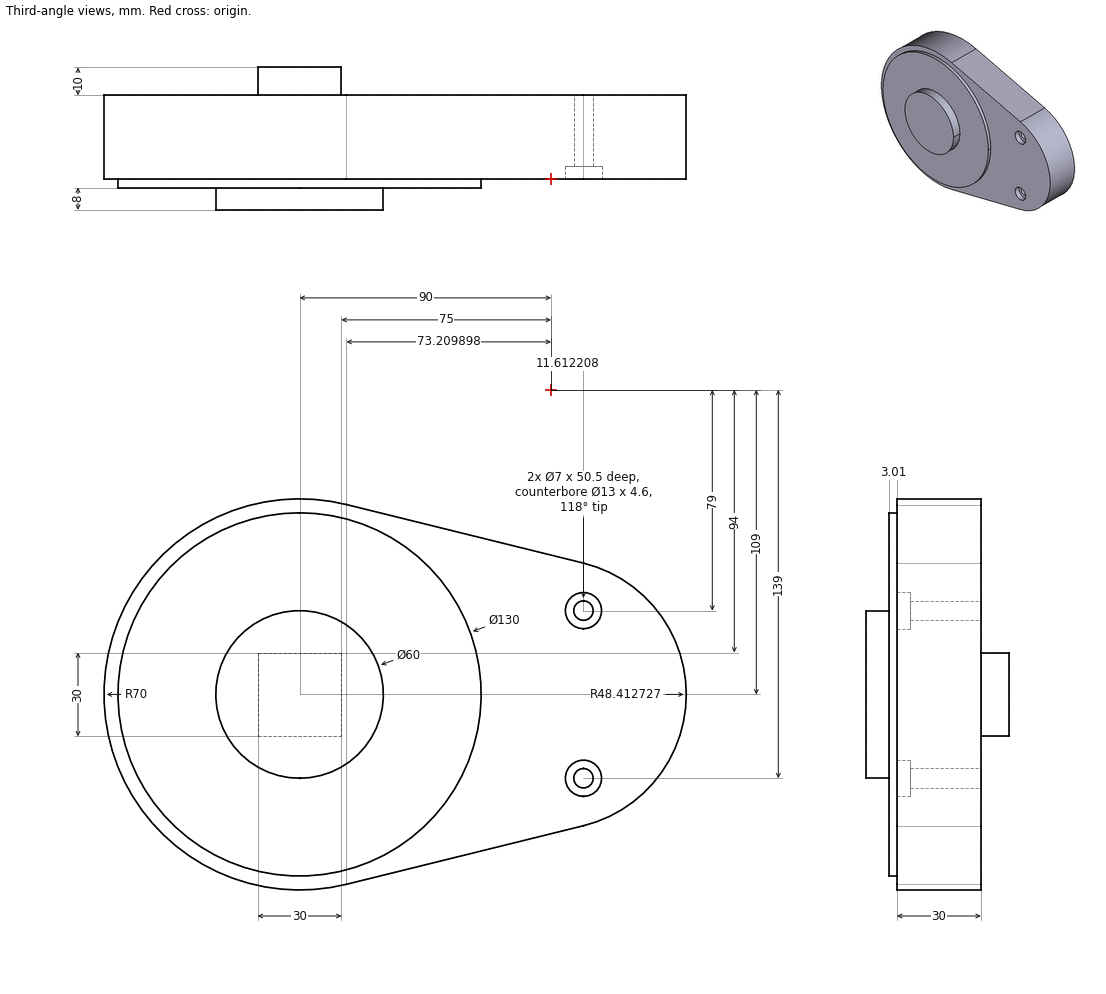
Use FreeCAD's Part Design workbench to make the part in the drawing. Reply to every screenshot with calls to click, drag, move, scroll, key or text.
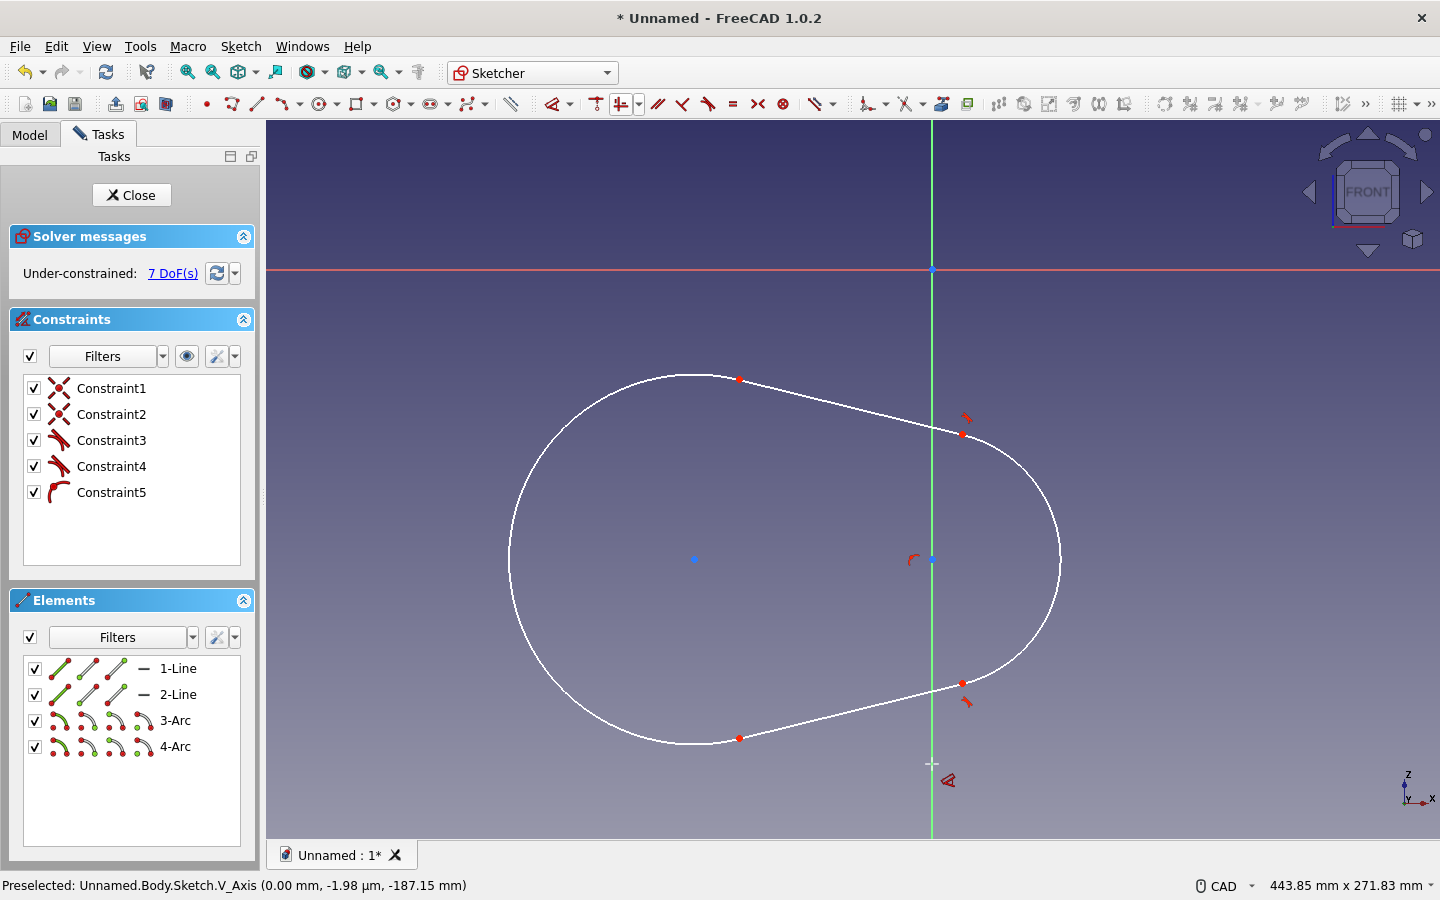
click(556, 437)
click(532, 416)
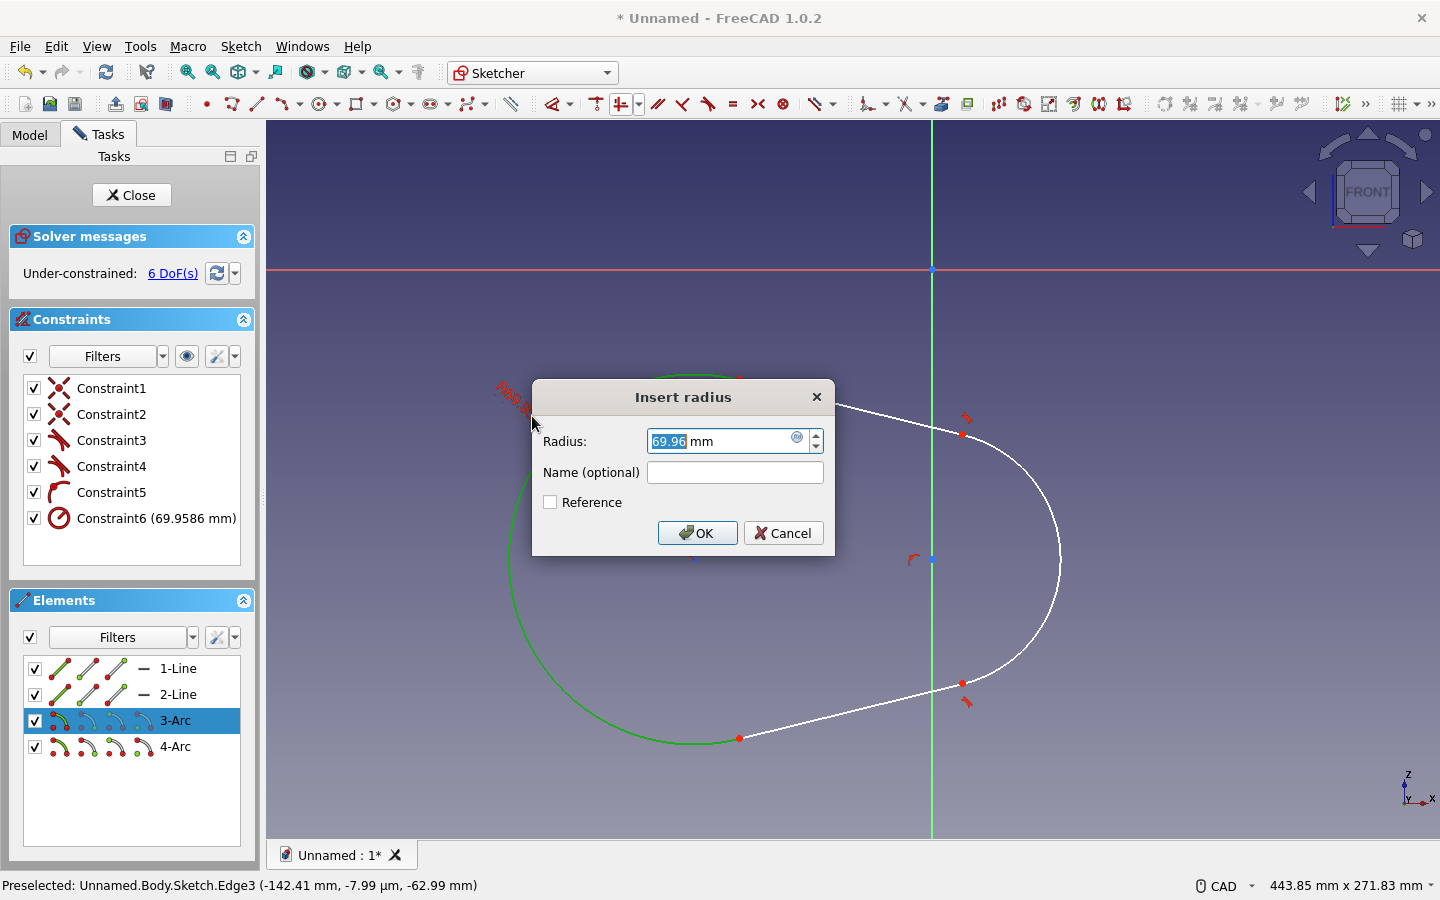
text(70)
key(Return)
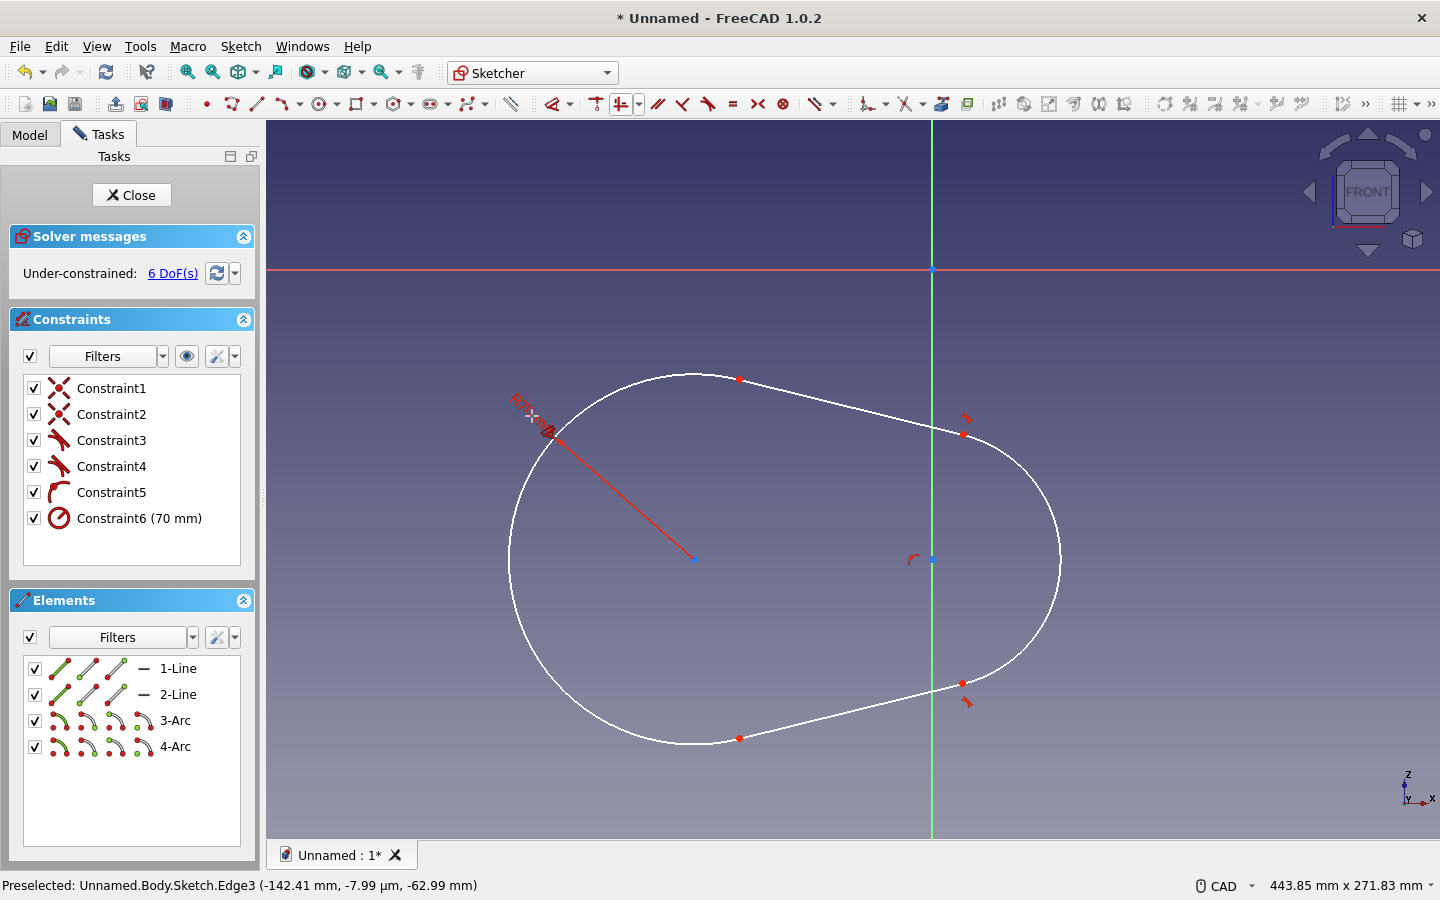
click(1043, 625)
click(1071, 641)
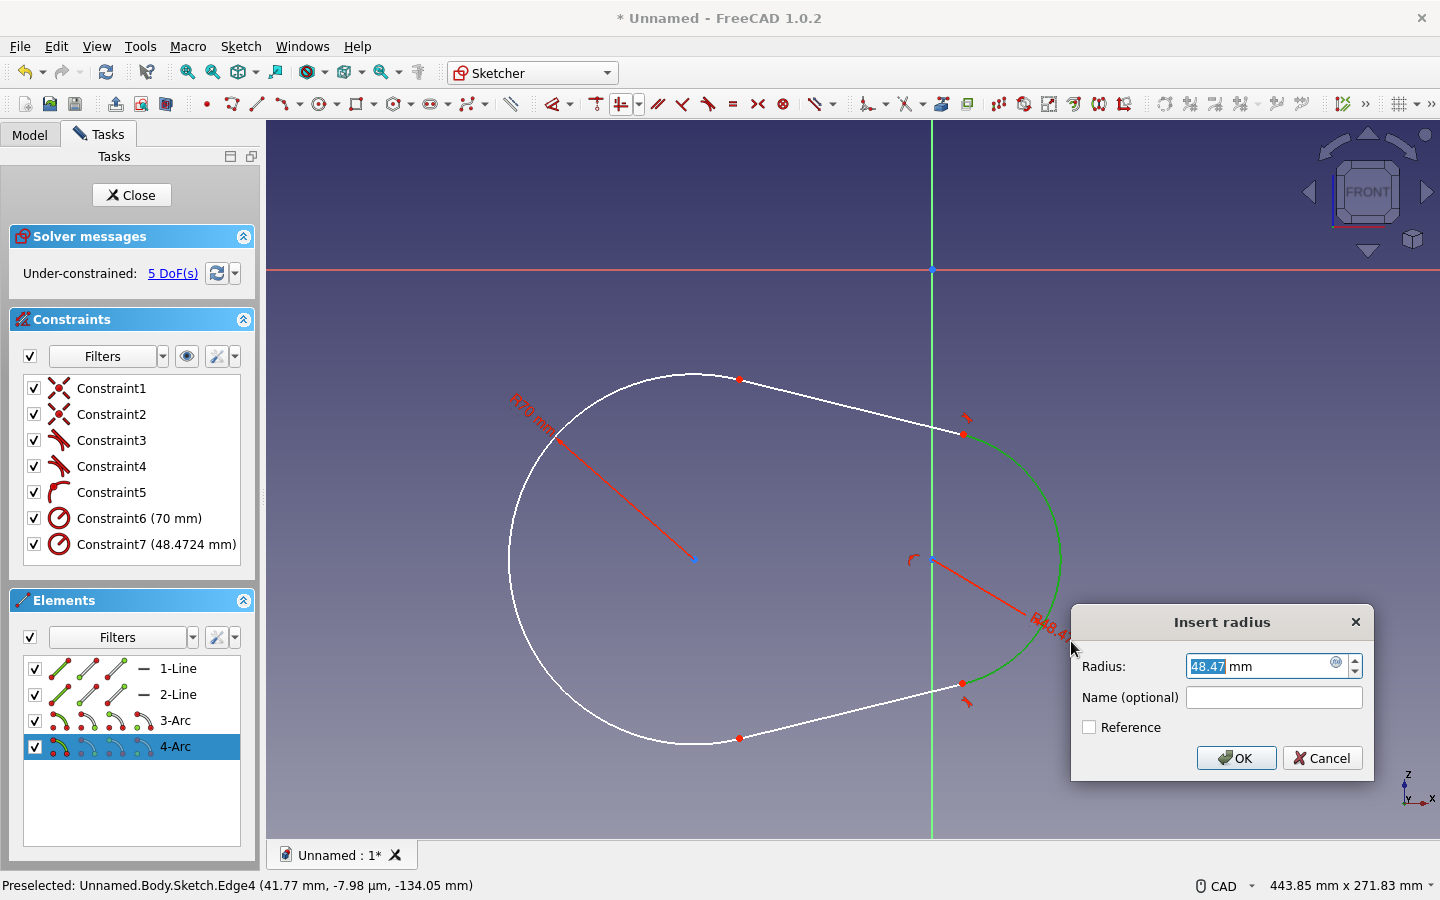
text(48.412727)
key(Return)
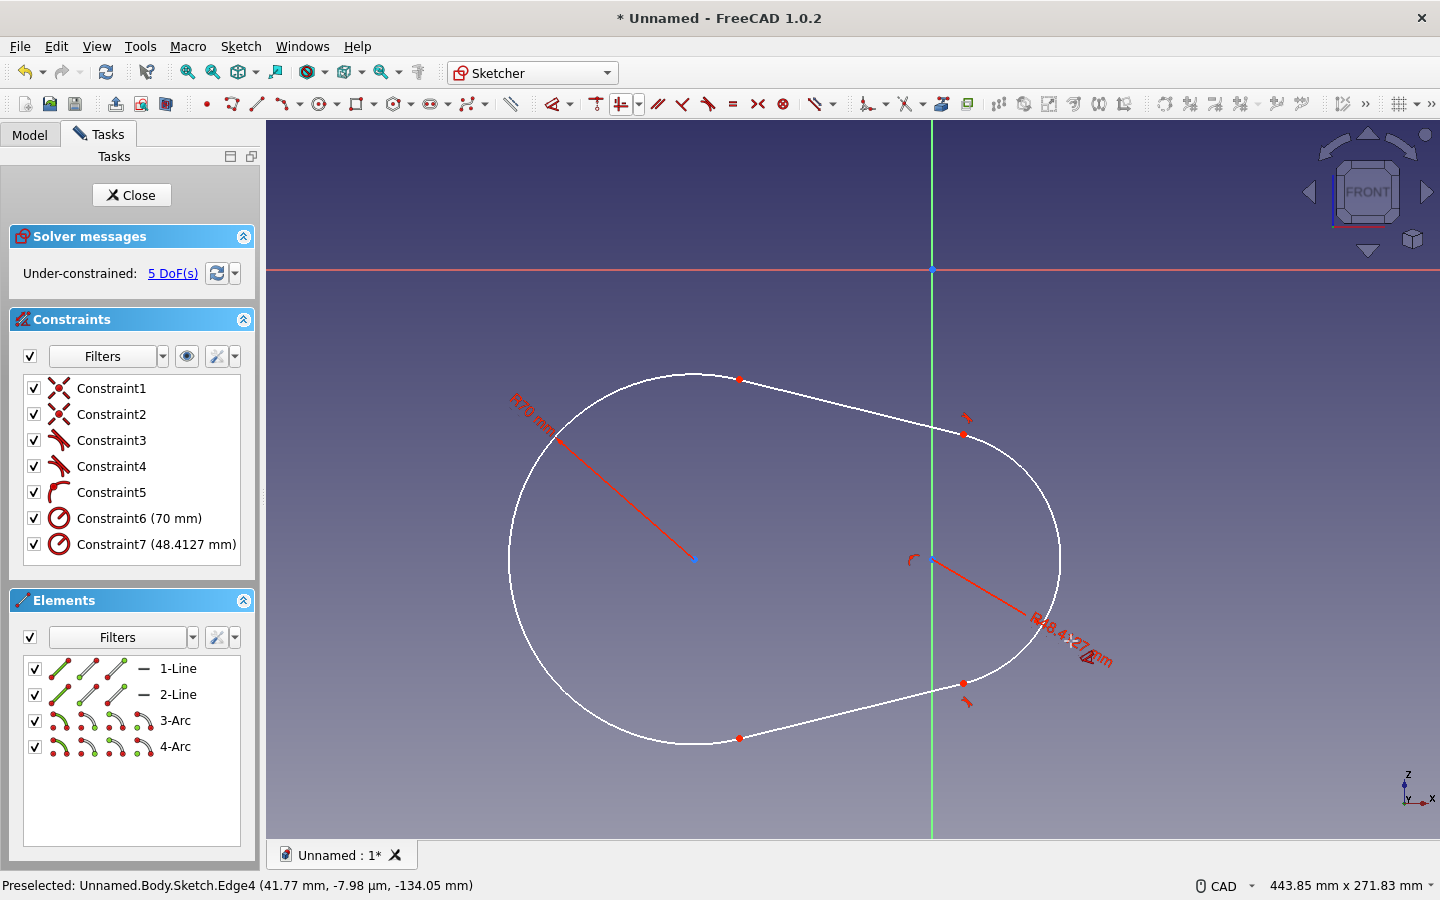
click(694, 559)
click(813, 236)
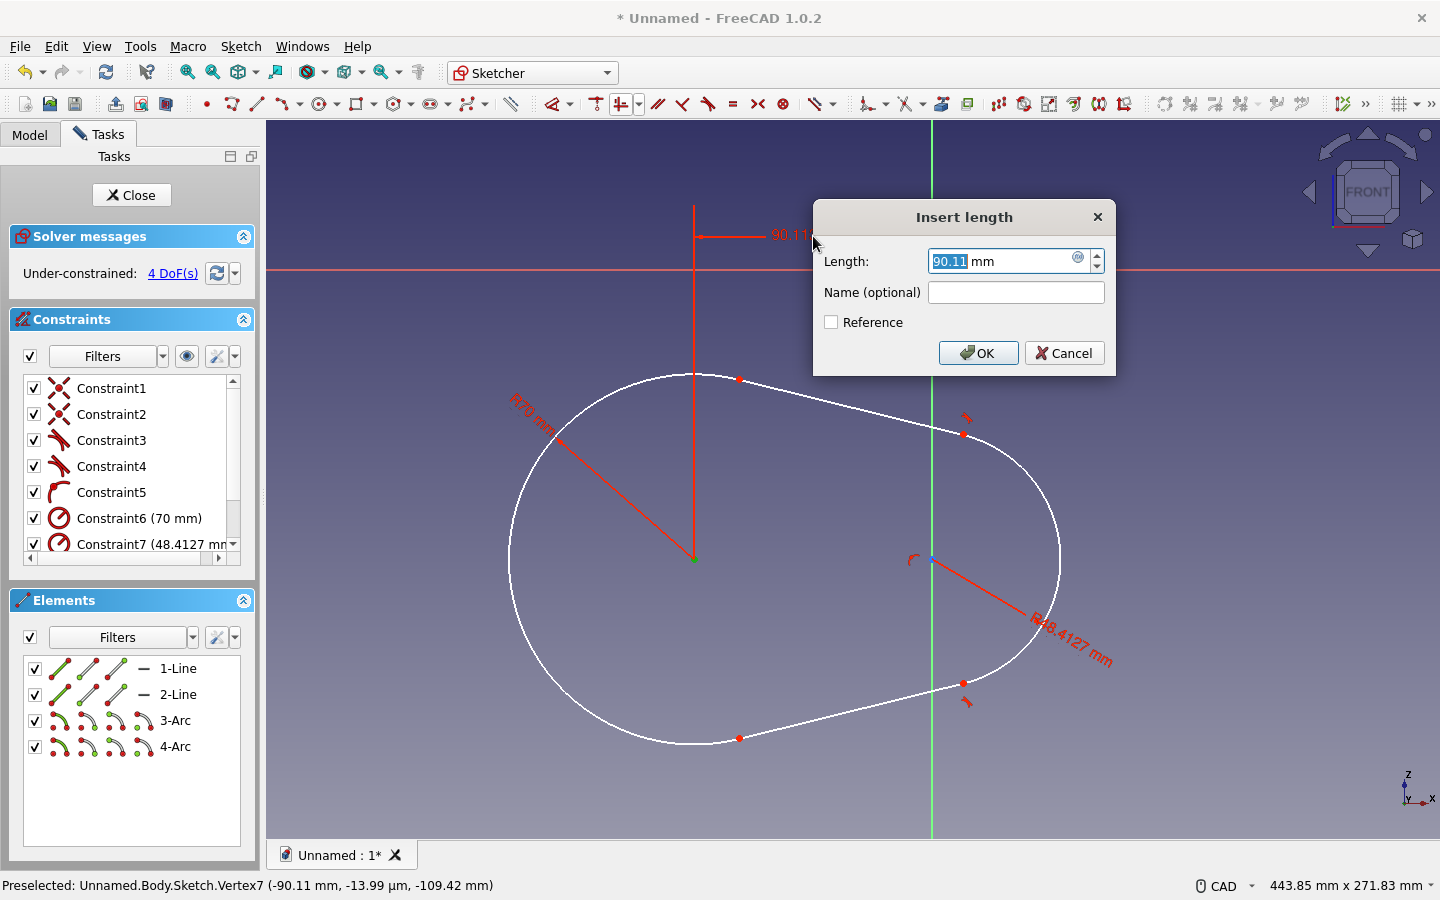
text(90)
key(Return)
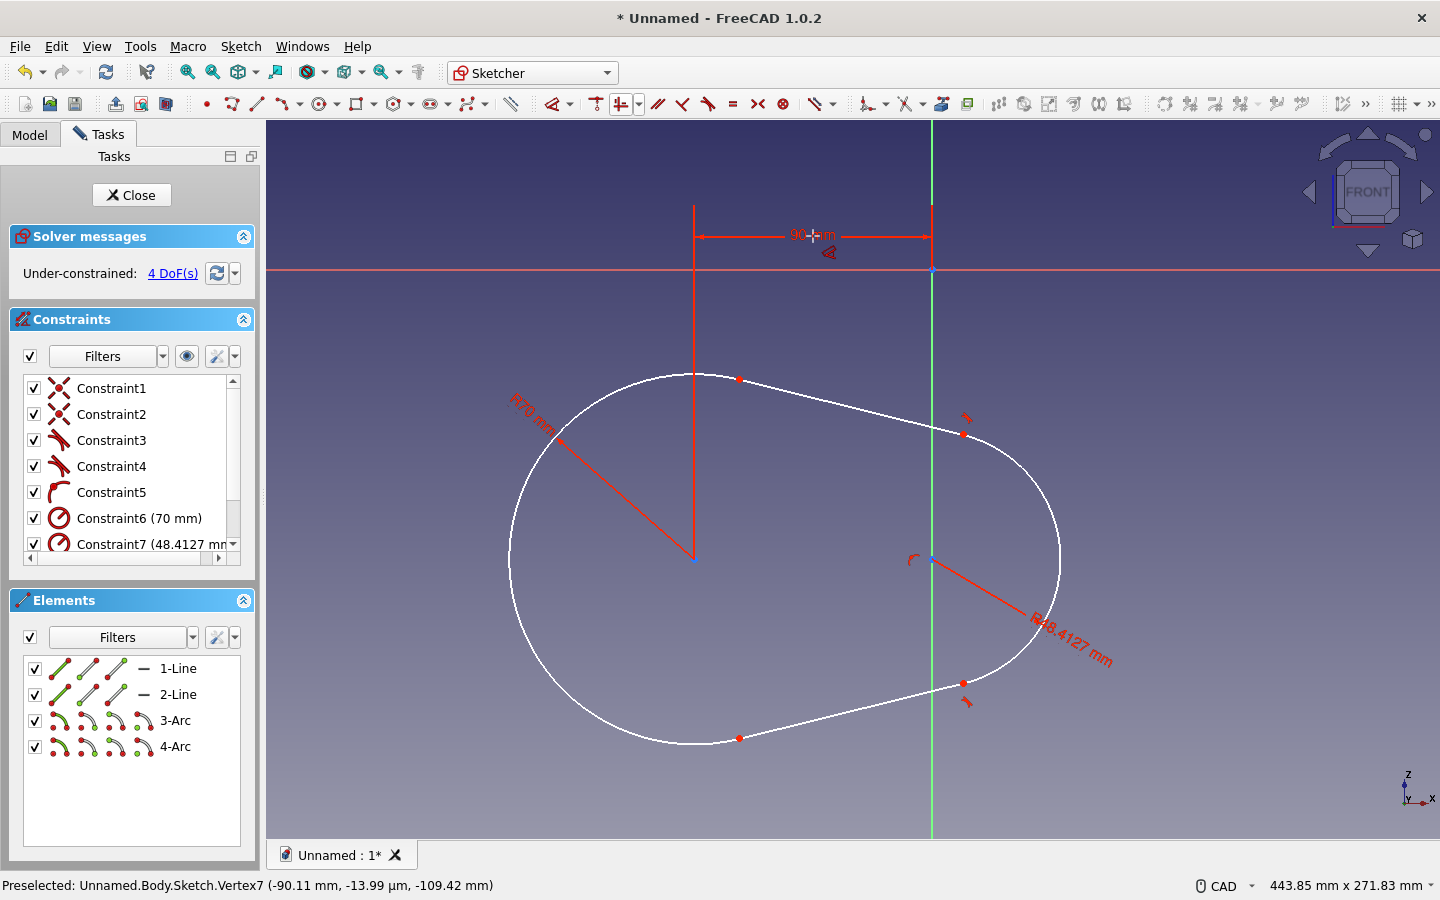
click(694, 559)
click(966, 415)